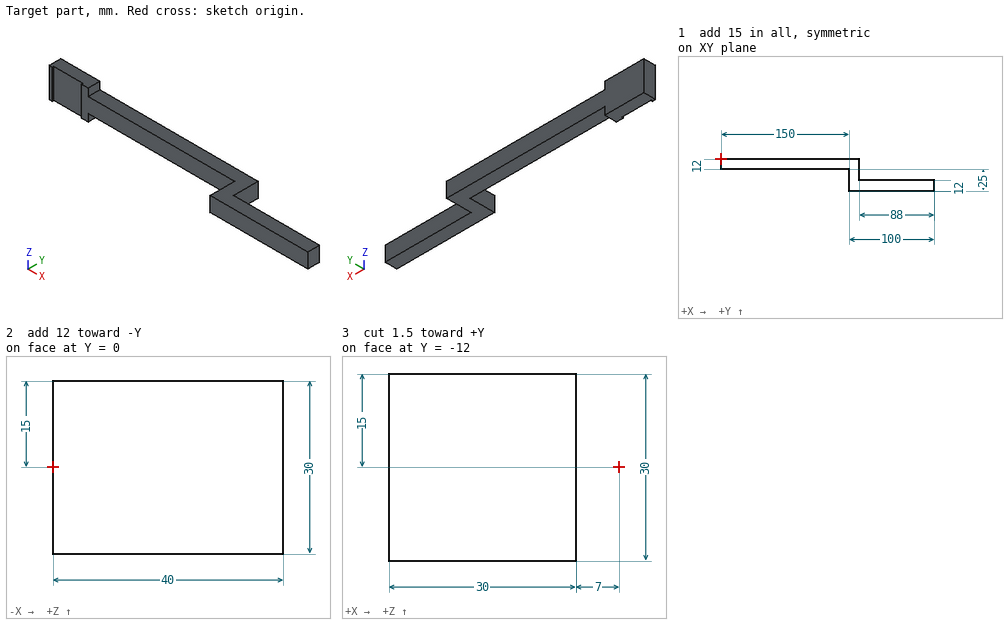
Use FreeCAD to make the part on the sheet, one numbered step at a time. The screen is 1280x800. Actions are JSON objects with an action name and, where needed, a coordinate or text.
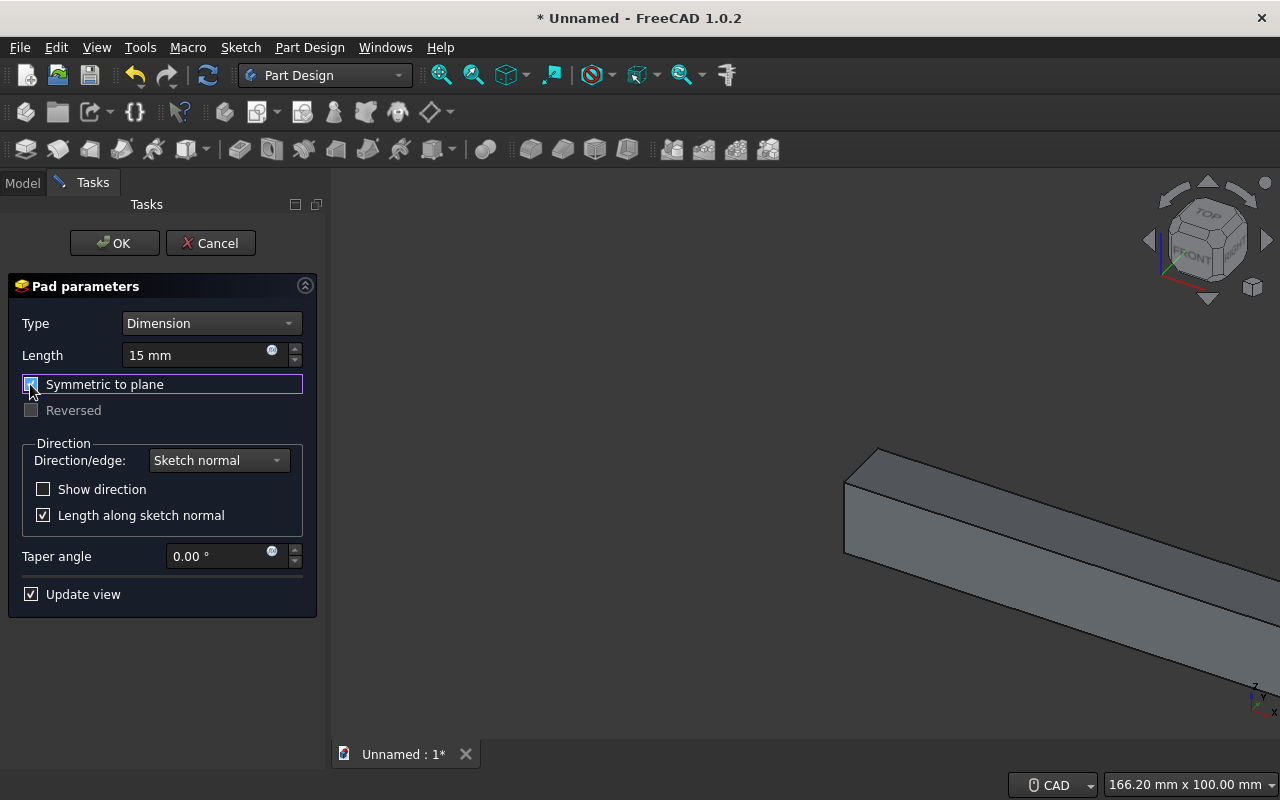
{"action": "left_click", "coordinate": [115, 243]}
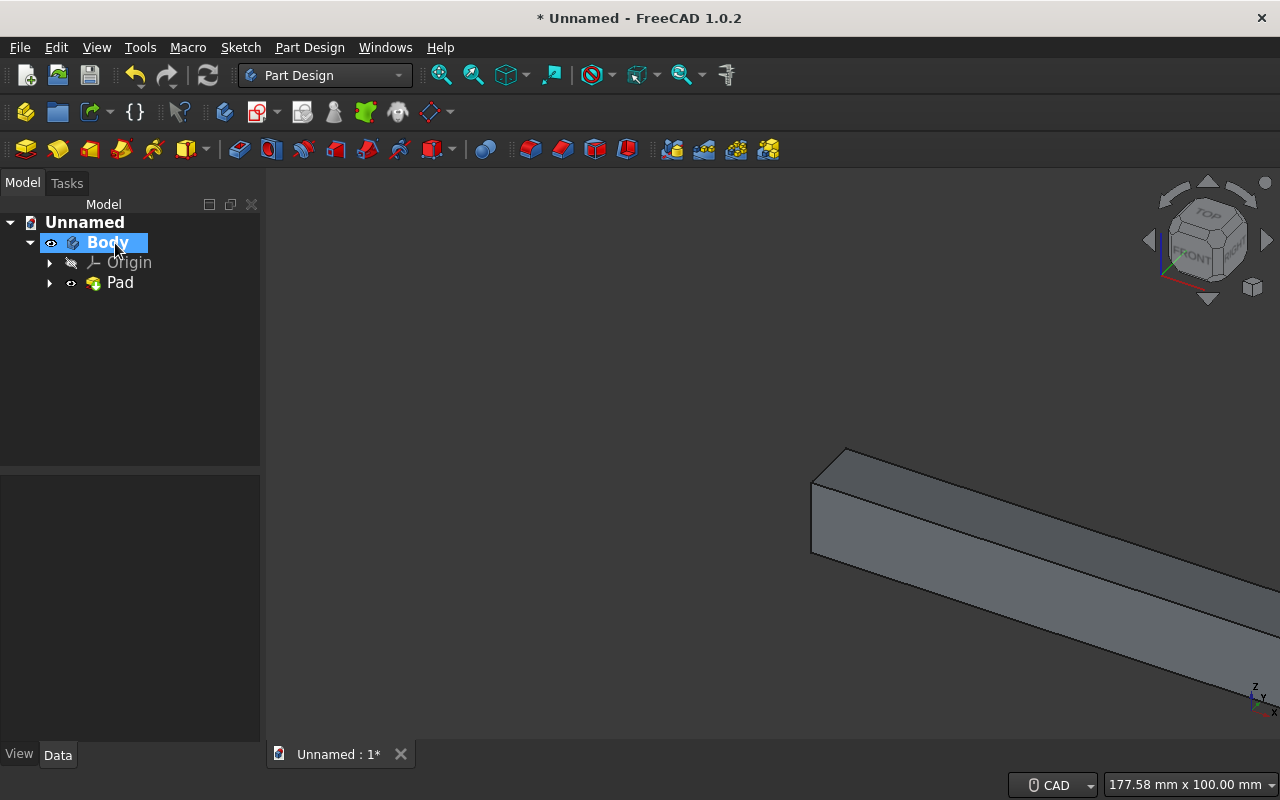
{"action": "left_click", "coordinate": [442, 76]}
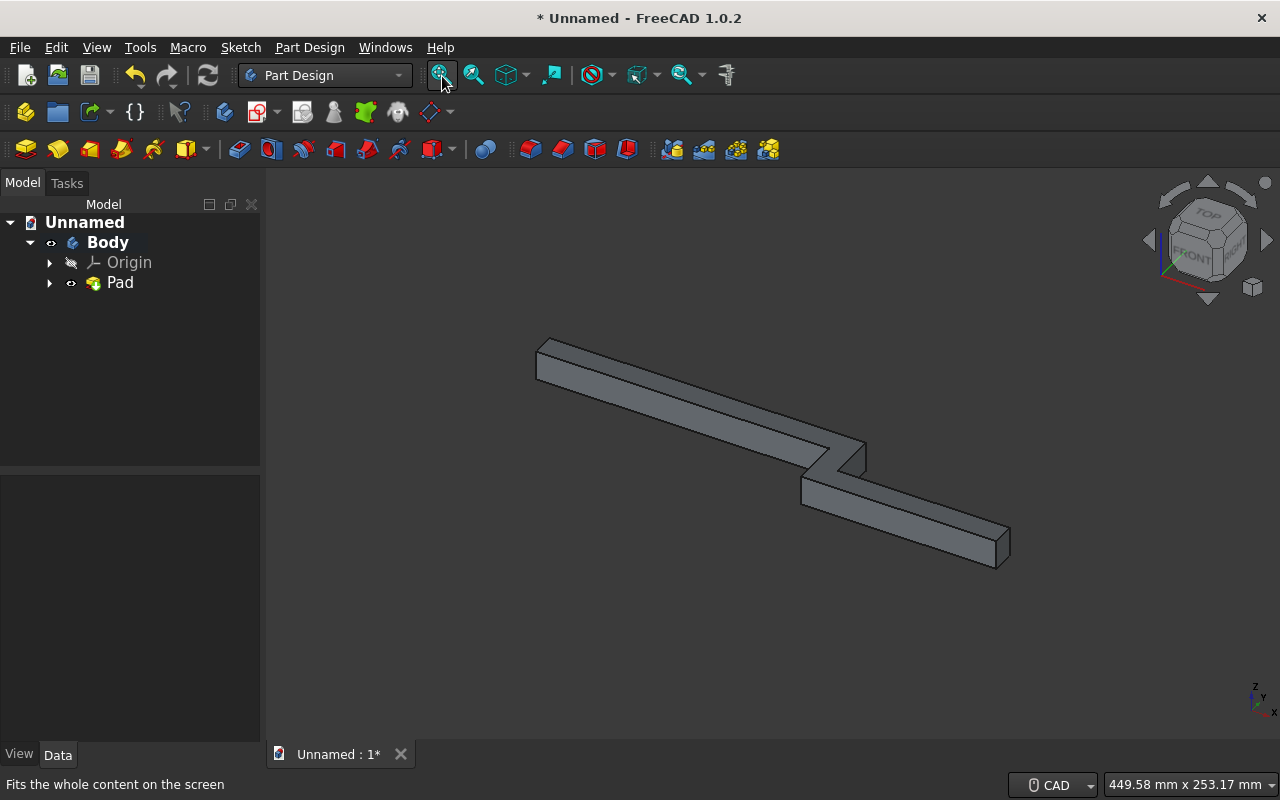
{"action": "key", "text": "4"}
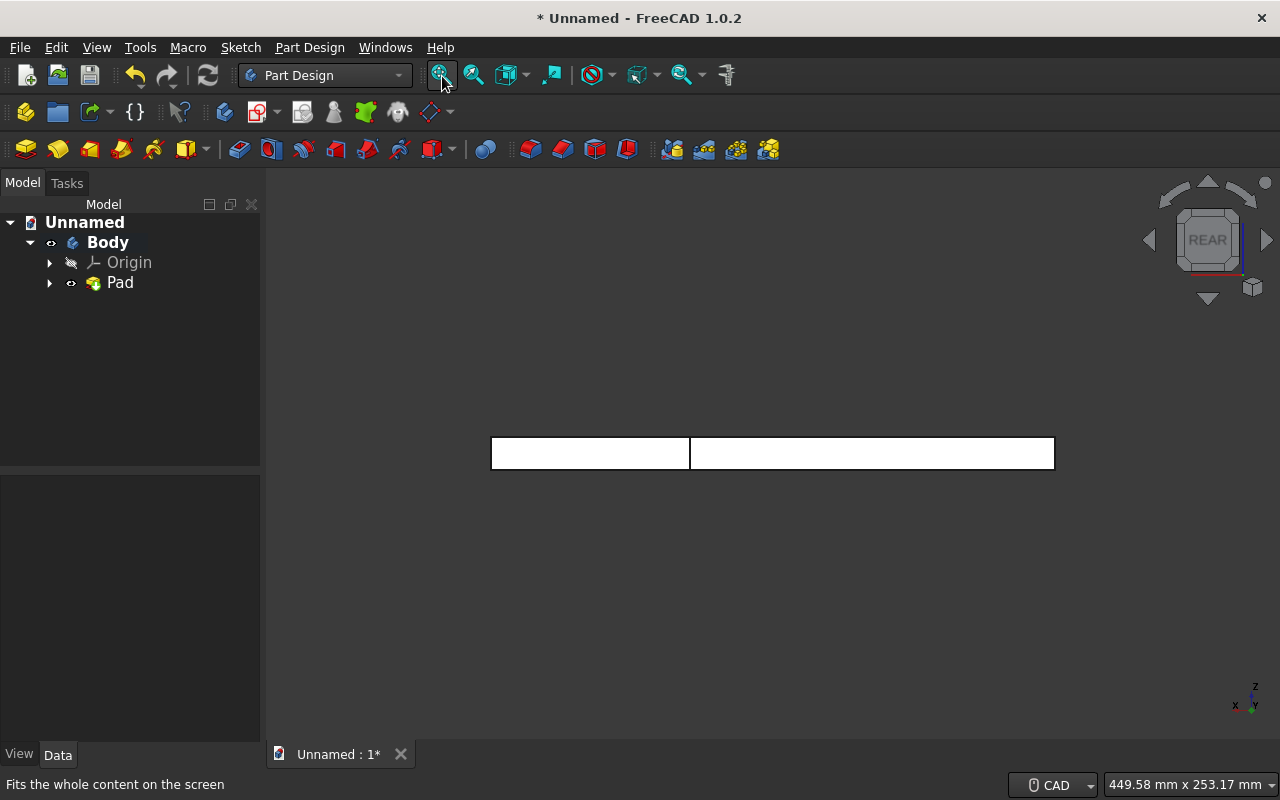
{"action": "left_click", "coordinate": [716, 452]}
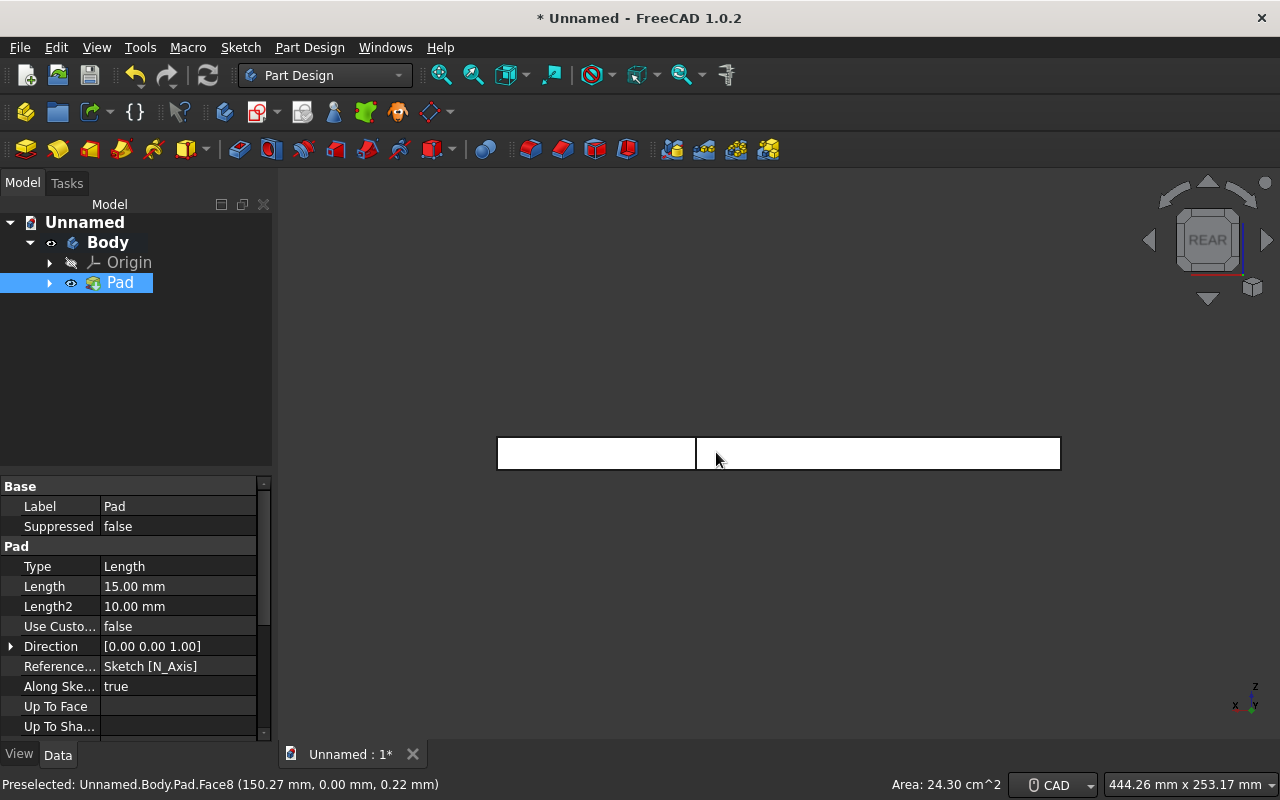
{"action": "left_click", "coordinate": [258, 112]}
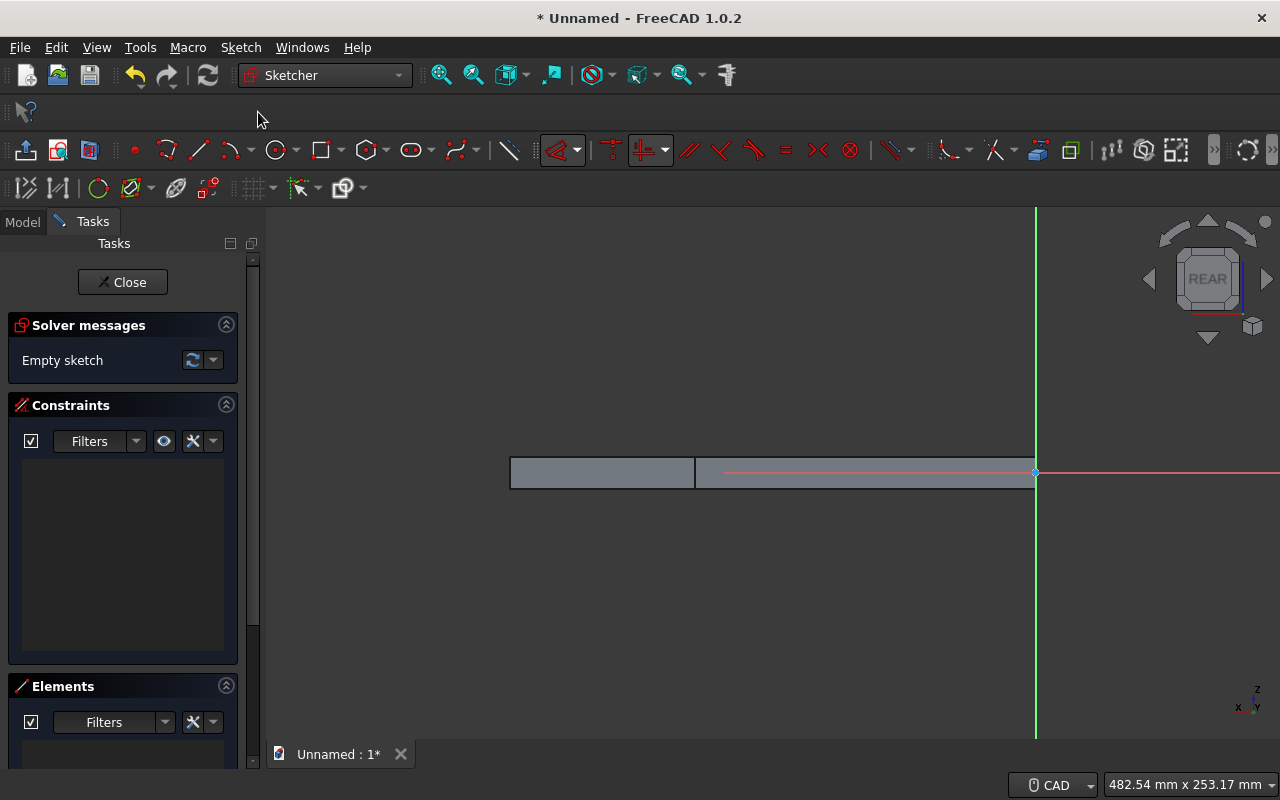
{"action": "scroll", "coordinate": [704, 473], "scroll_direction": "down", "scroll_amount": 5}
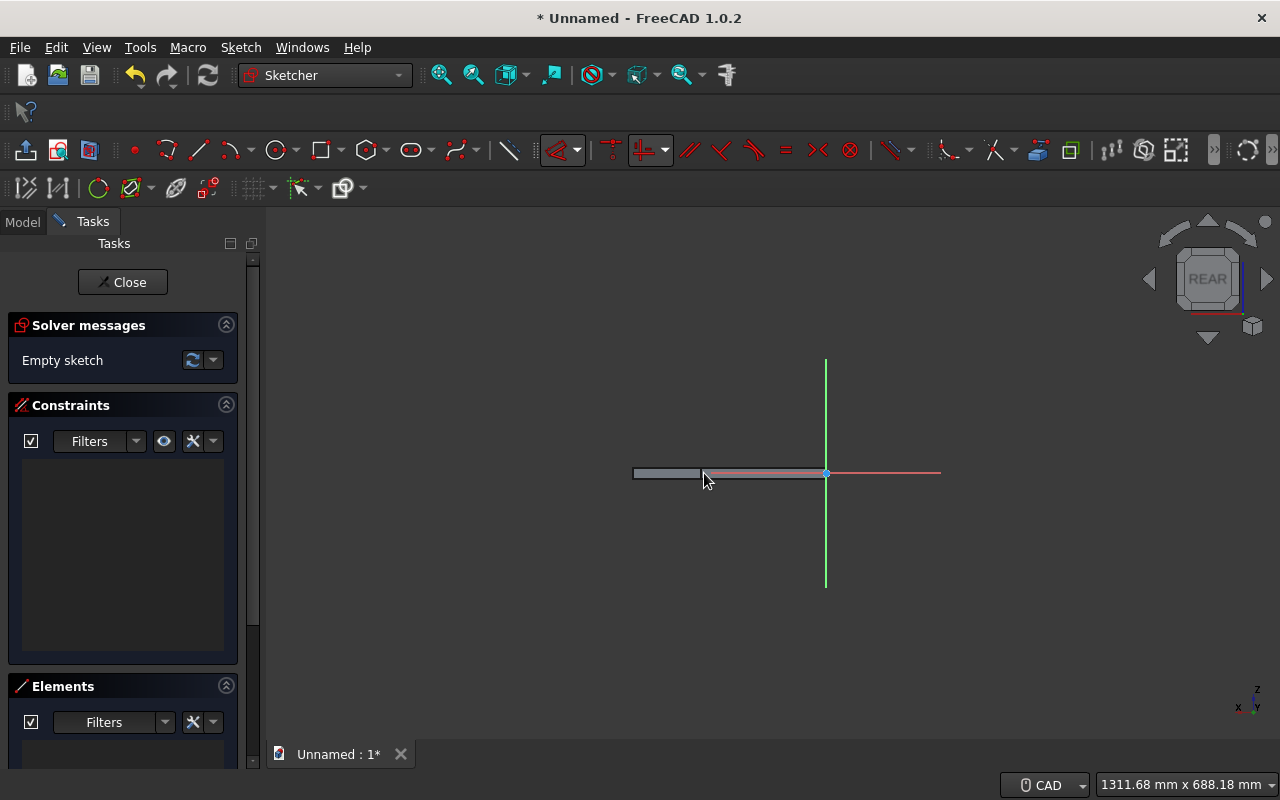
{"action": "scroll", "coordinate": [853, 473], "scroll_direction": "up", "scroll_amount": 13}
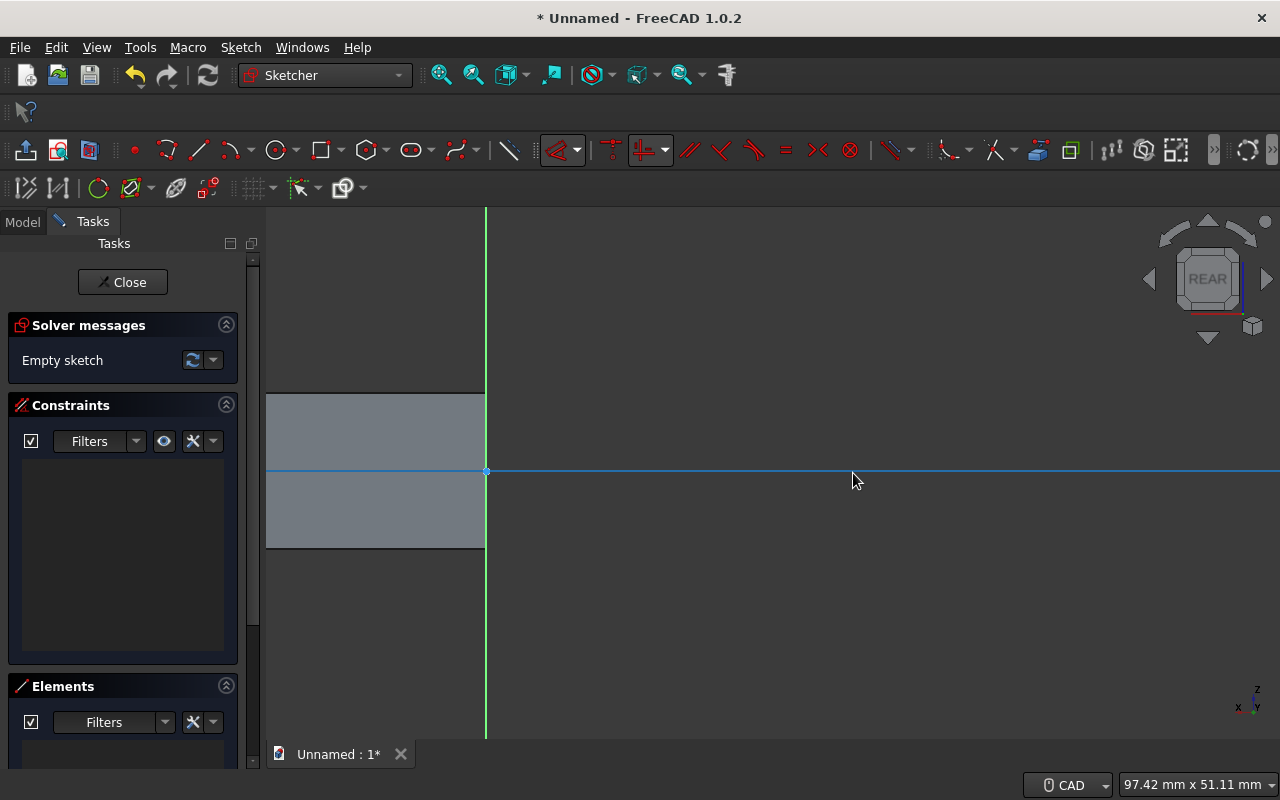
{"action": "left_click", "coordinate": [322, 150]}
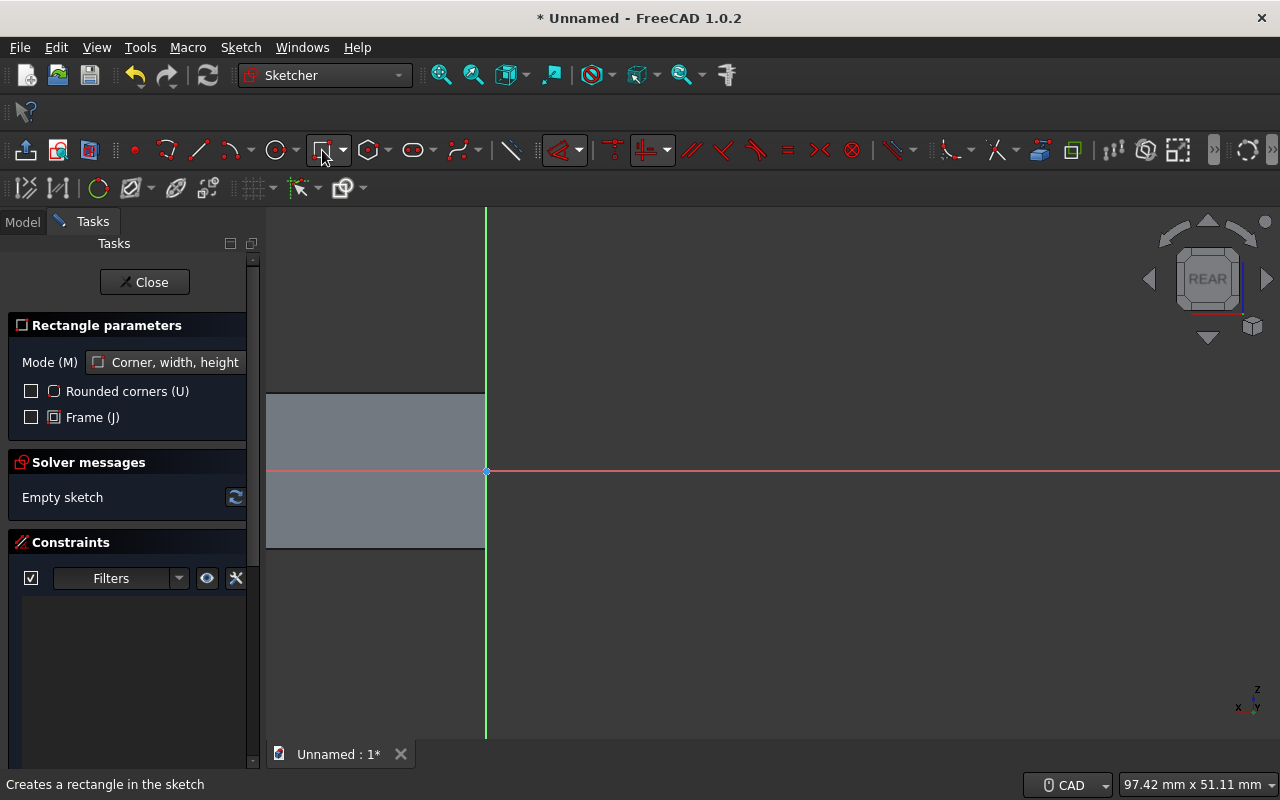
{"action": "left_click", "coordinate": [486, 315]}
{"action": "mouse_move", "coordinate": [902, 627]}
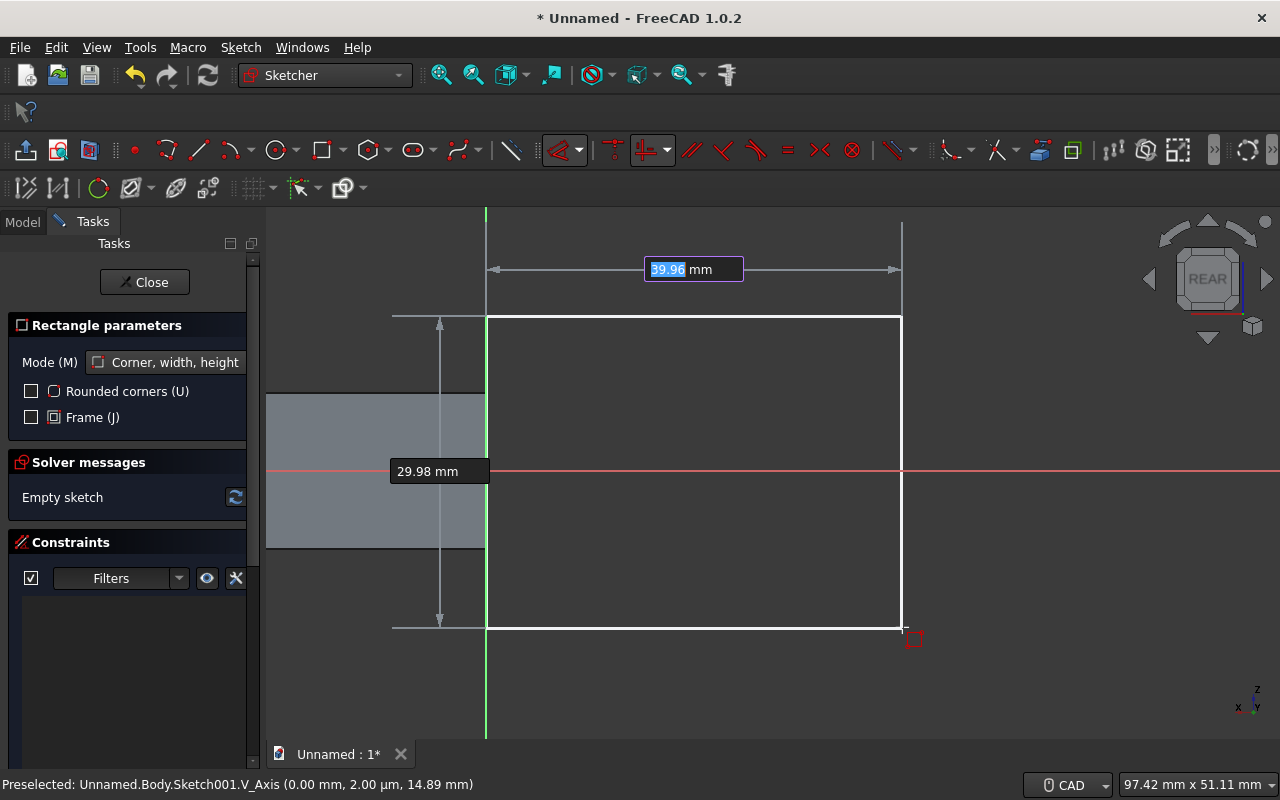
{"action": "type", "text": "40"}
{"action": "key", "text": "Tab"}
{"action": "type", "text": "30"}
{"action": "key", "text": "Return"}
{"action": "key", "text": "Escape"}